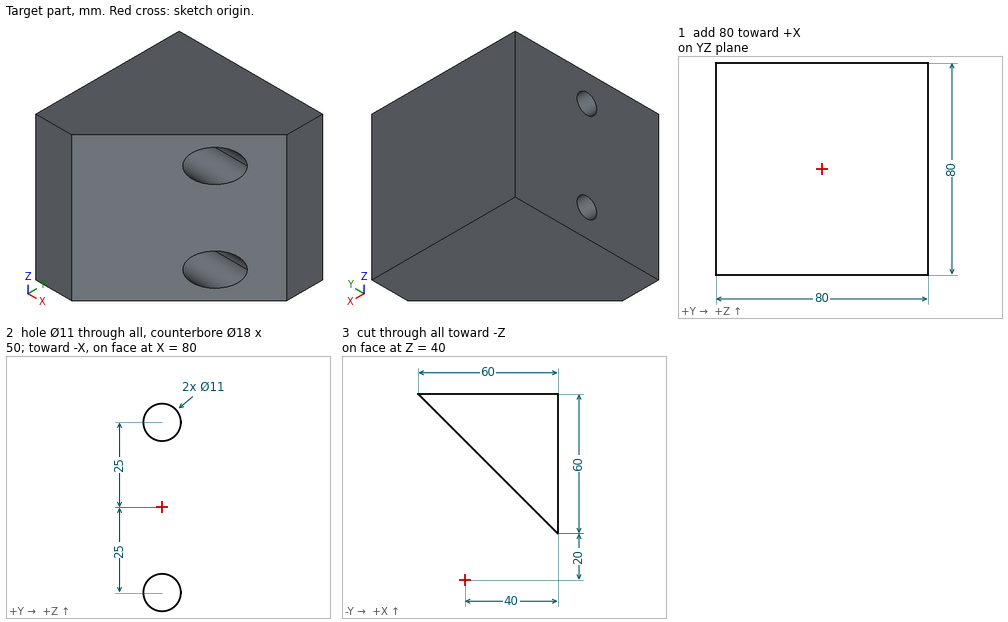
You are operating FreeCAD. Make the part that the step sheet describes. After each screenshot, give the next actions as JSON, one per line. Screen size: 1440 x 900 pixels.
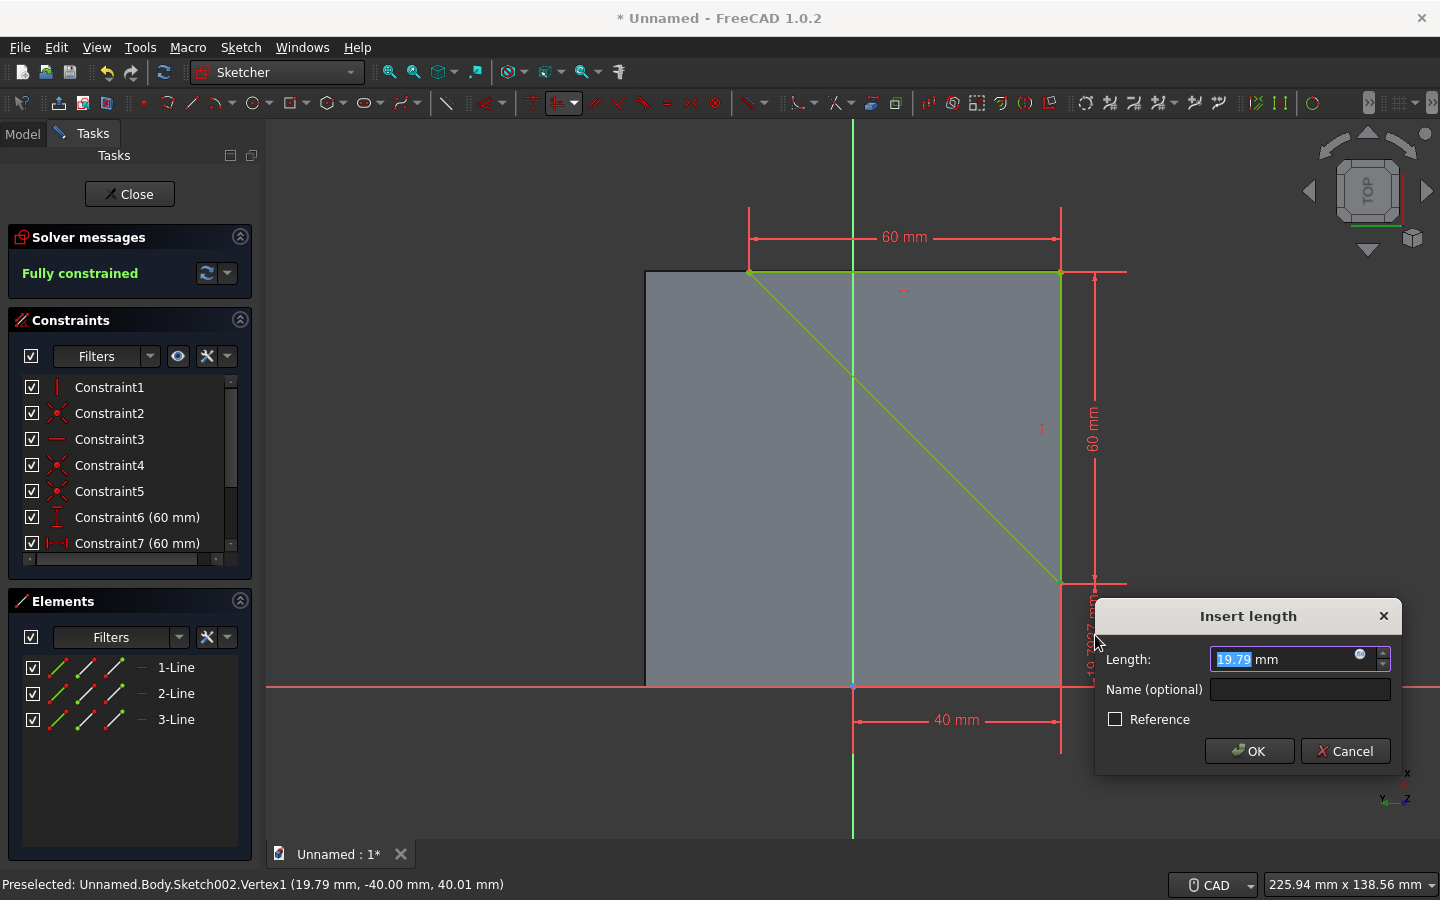
{"action": "type", "text": "20"}
{"action": "key", "text": "Return"}
{"action": "key", "text": "Escape"}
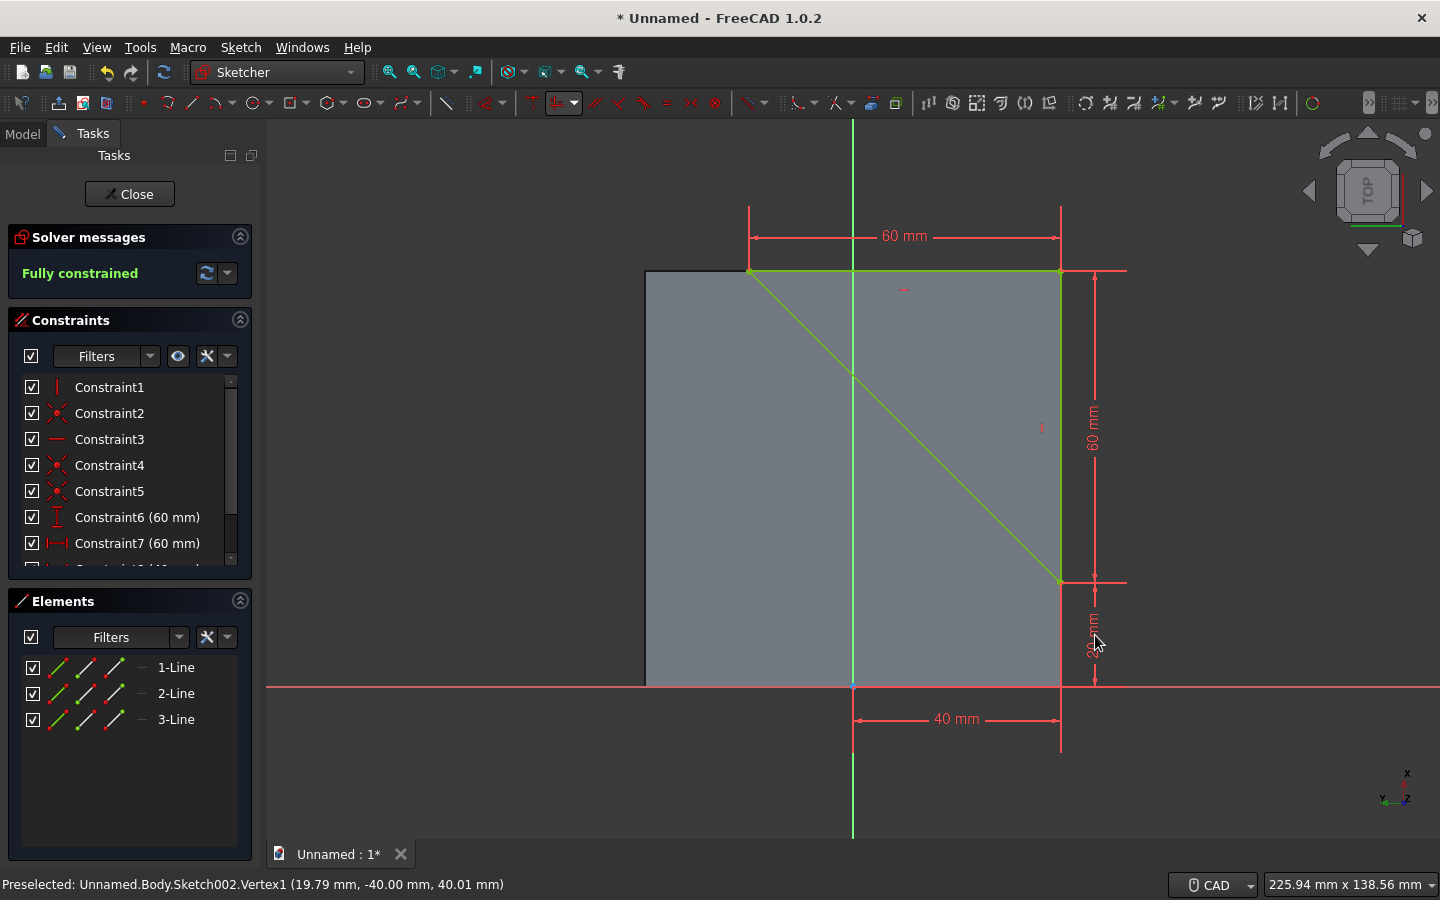
{"action": "left_click", "coordinate": [130, 194]}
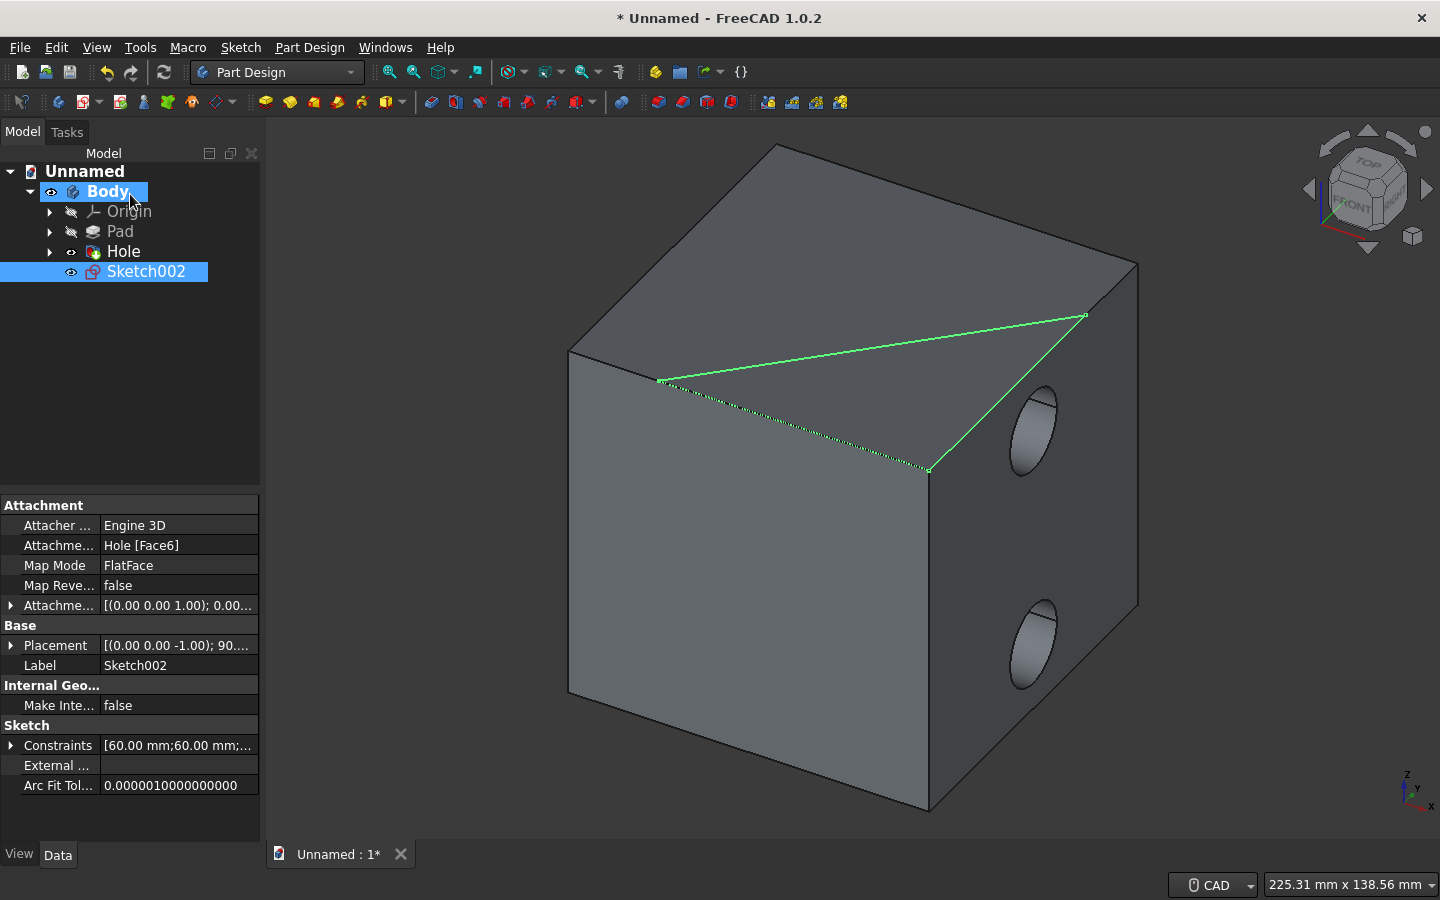
{"action": "left_click", "coordinate": [432, 102]}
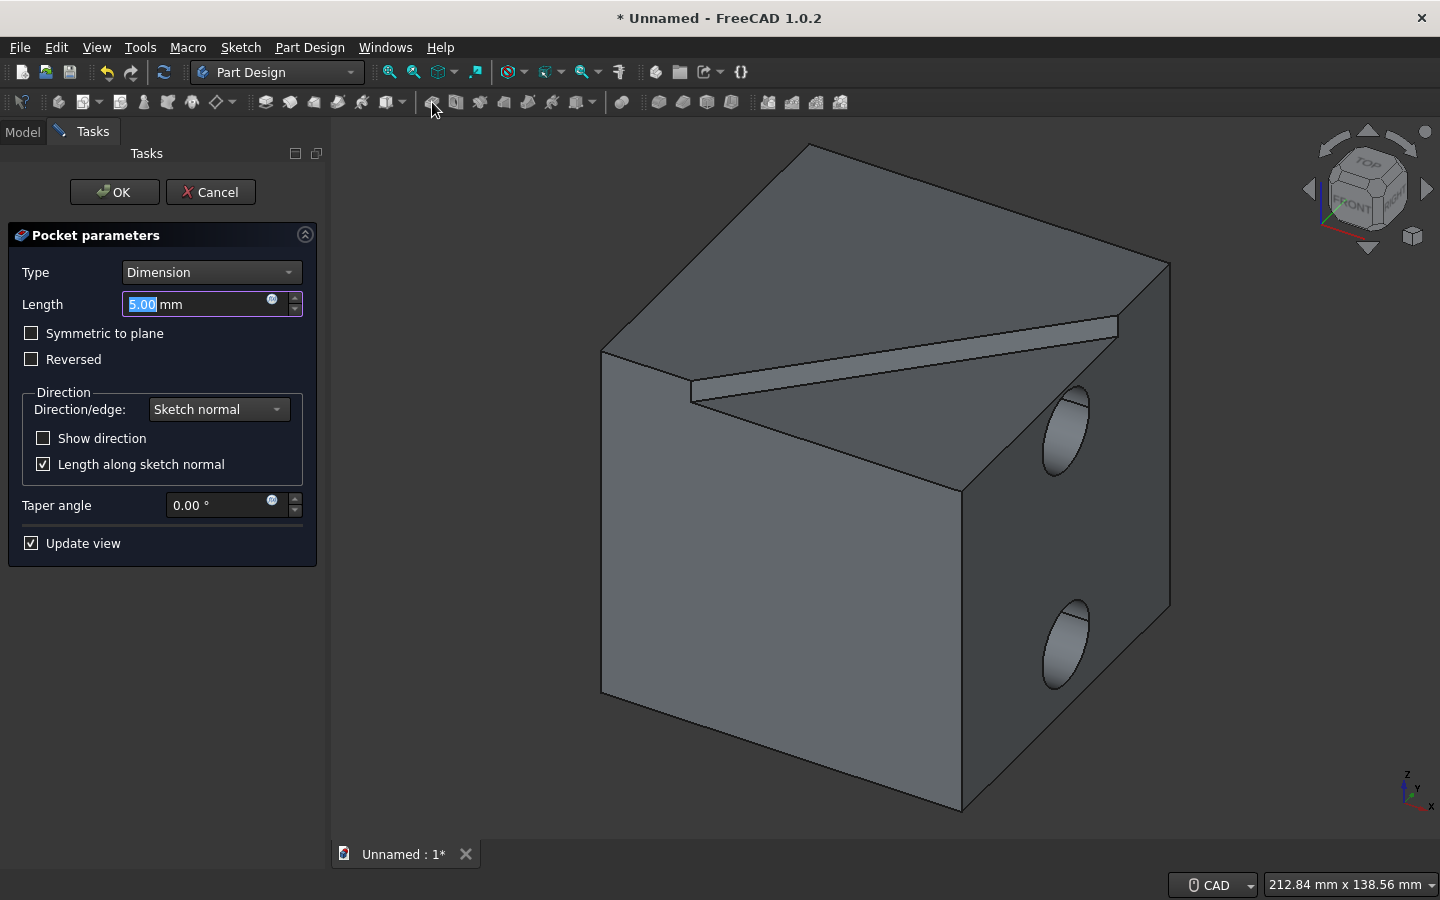
{"action": "left_click", "coordinate": [212, 272]}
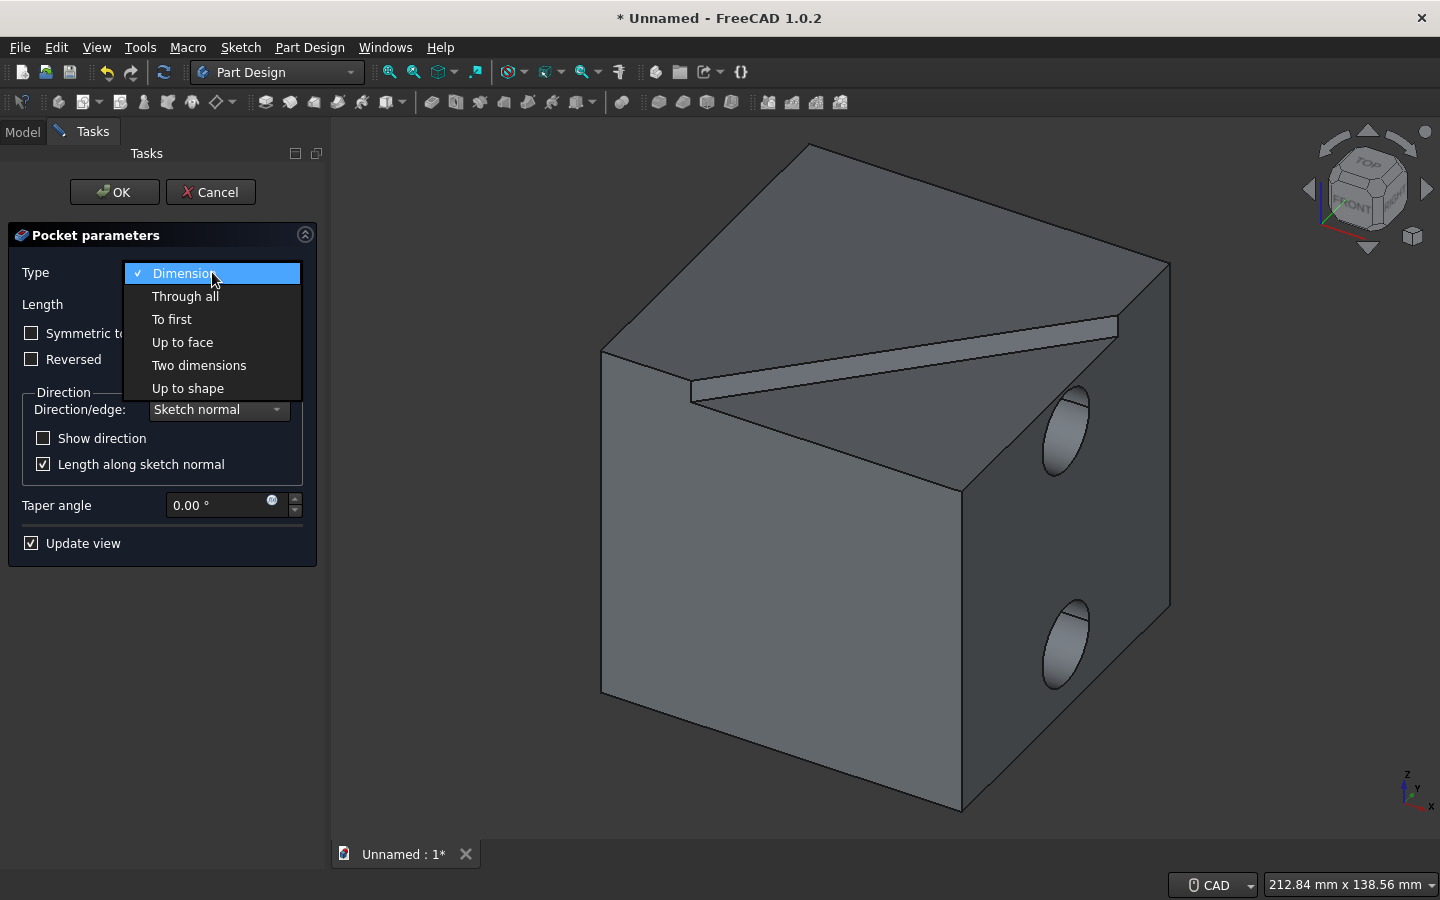
{"action": "left_click", "coordinate": [212, 296]}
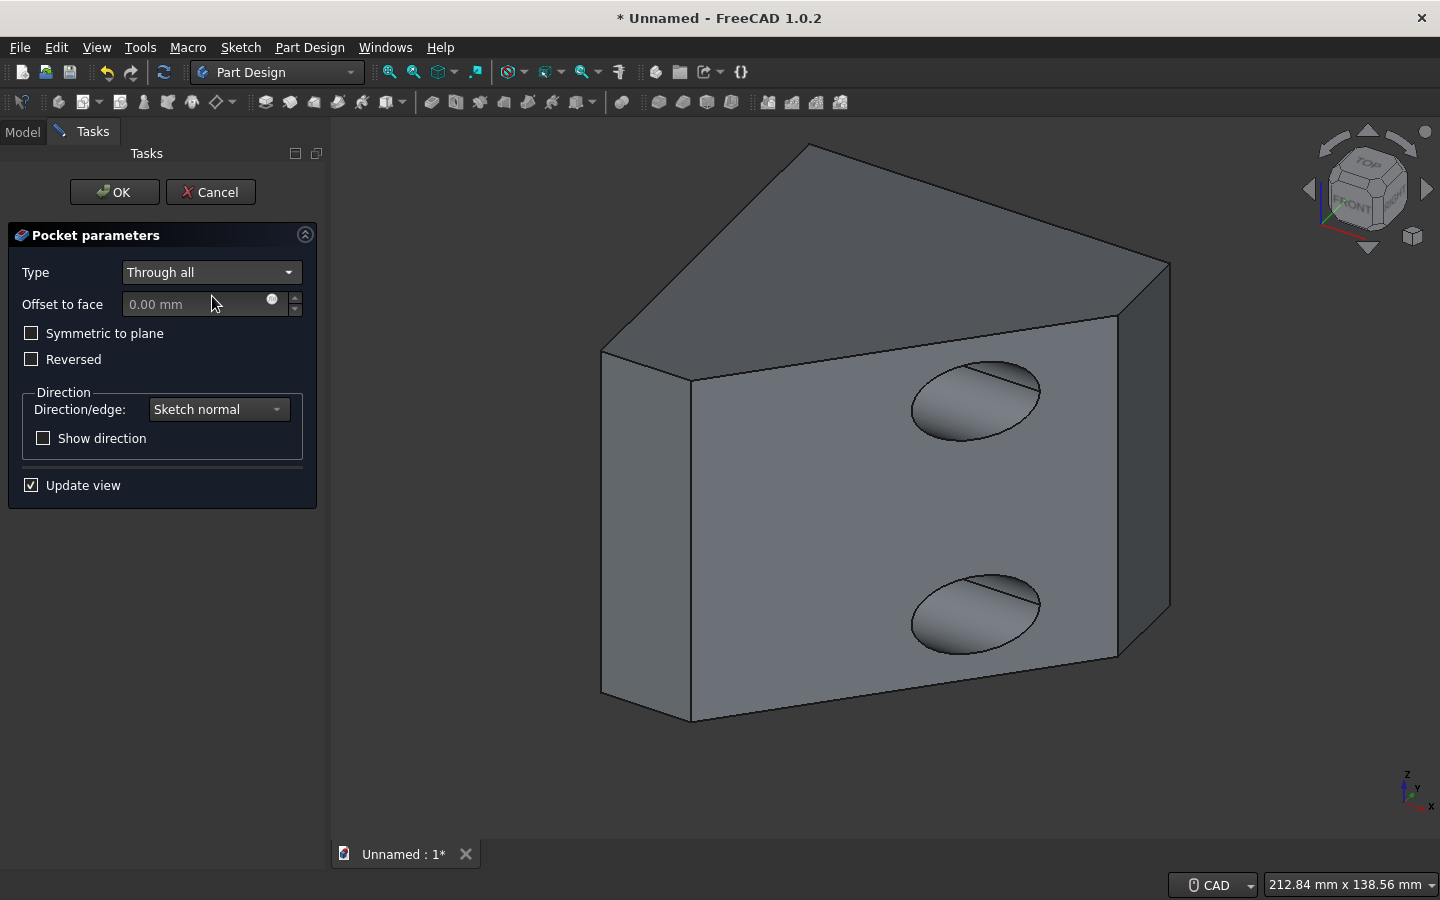
{"action": "left_click", "coordinate": [115, 192]}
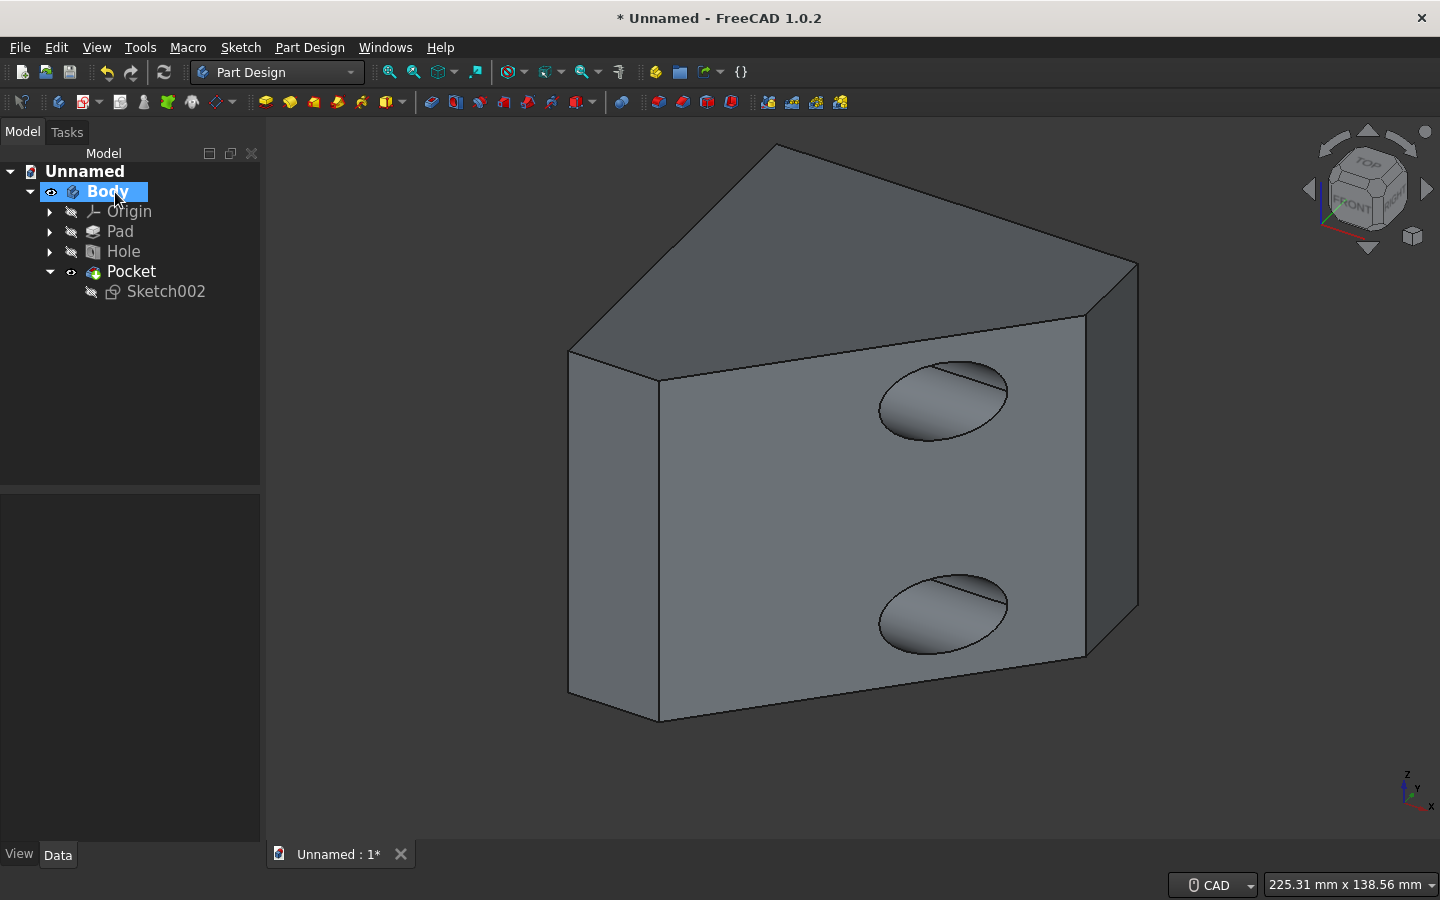
{"action": "key", "text": "0"}